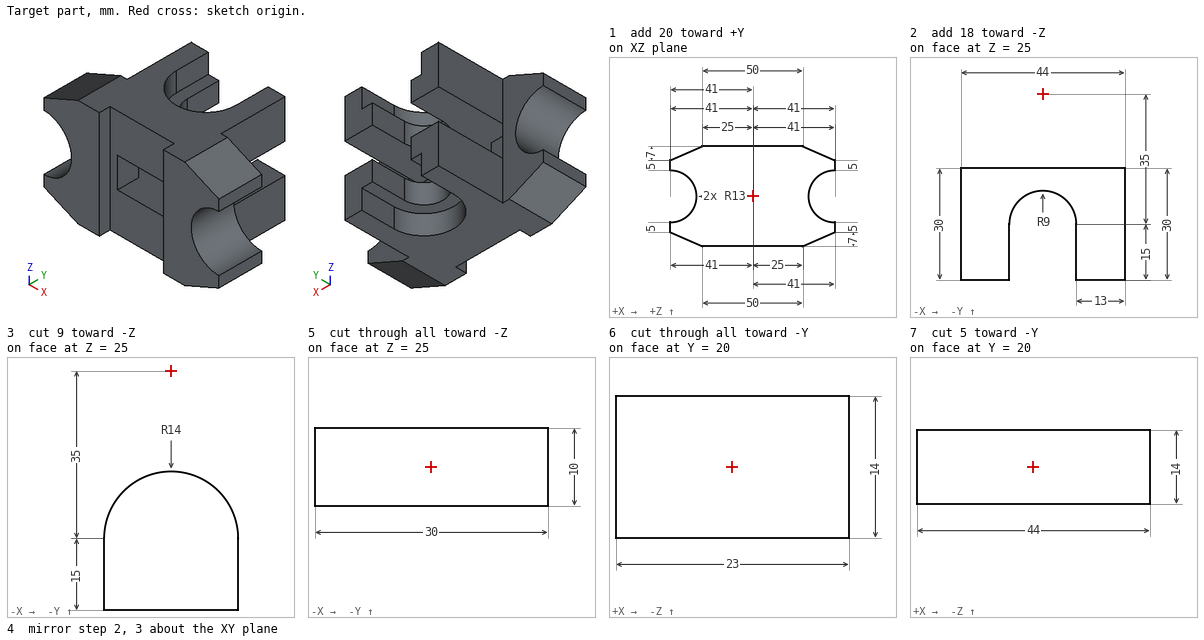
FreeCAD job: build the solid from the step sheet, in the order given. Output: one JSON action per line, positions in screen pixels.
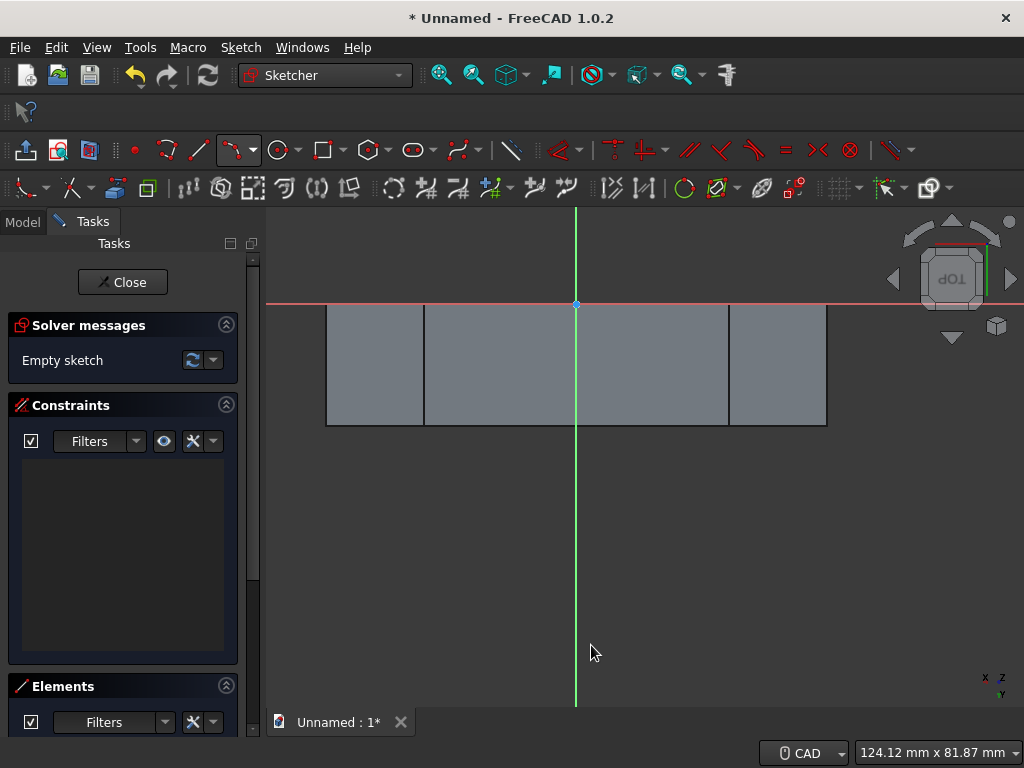
{"action": "left_click", "coordinate": [168, 150]}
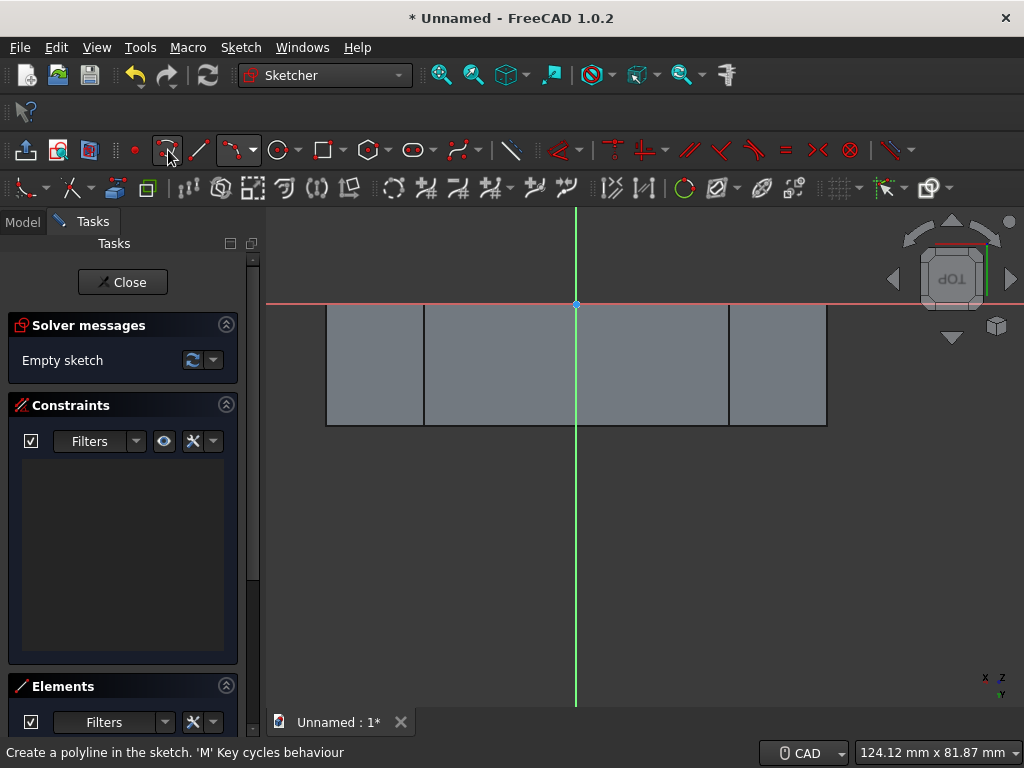
{"action": "left_click", "coordinate": [631, 518]}
{"action": "left_click", "coordinate": [631, 609]}
{"action": "left_click", "coordinate": [711, 609]}
{"action": "left_click", "coordinate": [711, 426]}
{"action": "left_click", "coordinate": [442, 426]}
{"action": "left_click", "coordinate": [442, 609]}
{"action": "left_click", "coordinate": [521, 609]}
{"action": "left_click", "coordinate": [521, 518]}
{"action": "right_click", "coordinate": [521, 518]}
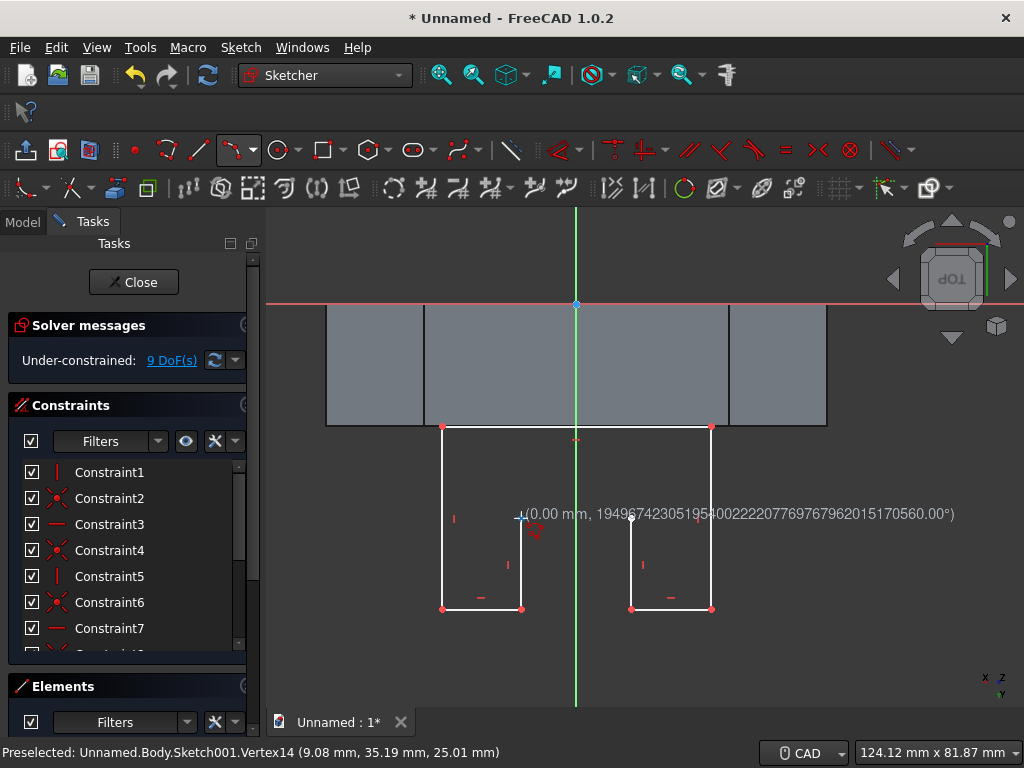
{"action": "left_click", "coordinate": [232, 150]}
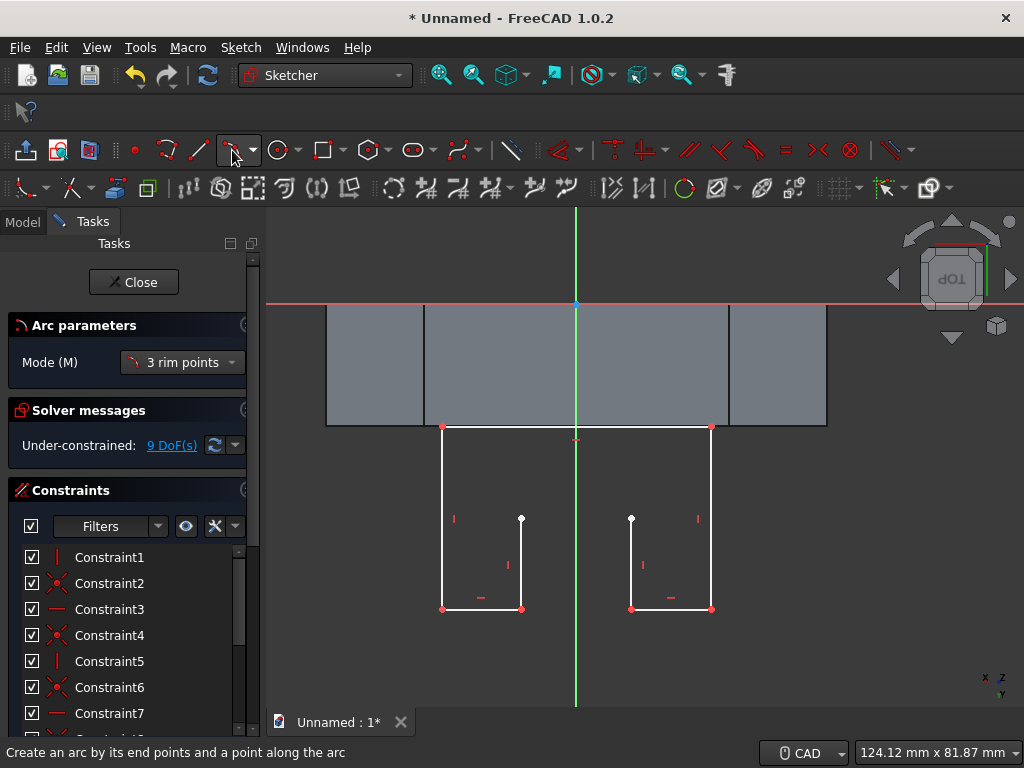
{"action": "left_click", "coordinate": [521, 519]}
{"action": "left_click", "coordinate": [631, 519]}
{"action": "left_click", "coordinate": [593, 466]}
{"action": "key", "text": "Escape"}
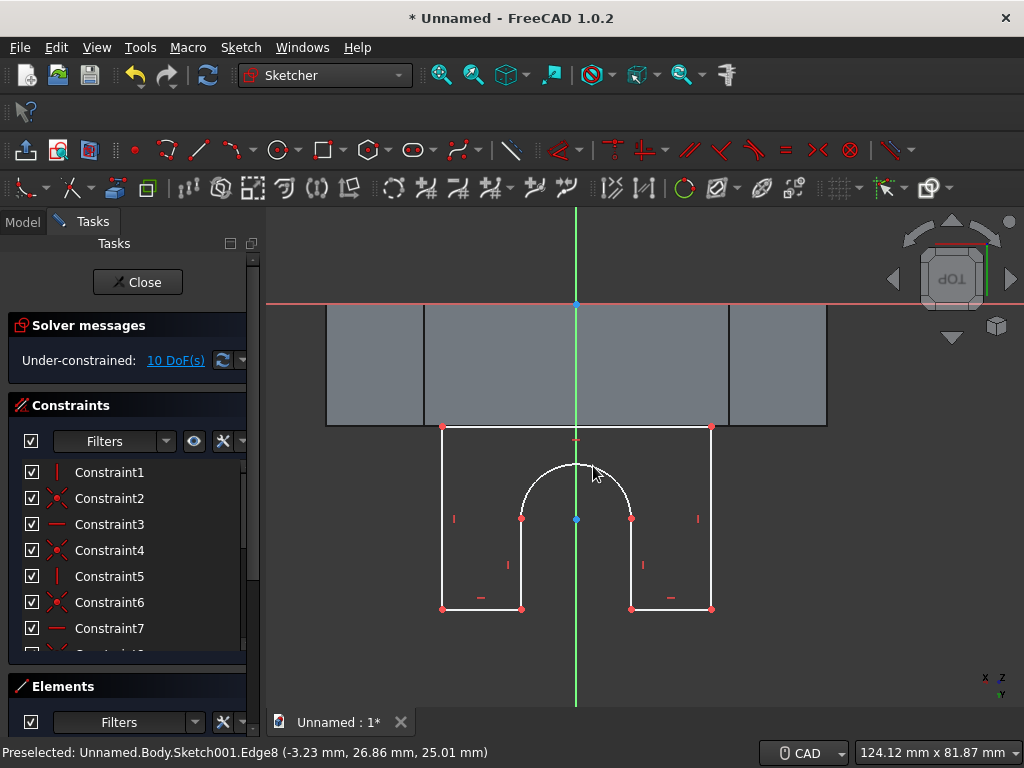
{"action": "left_click", "coordinate": [631, 546]}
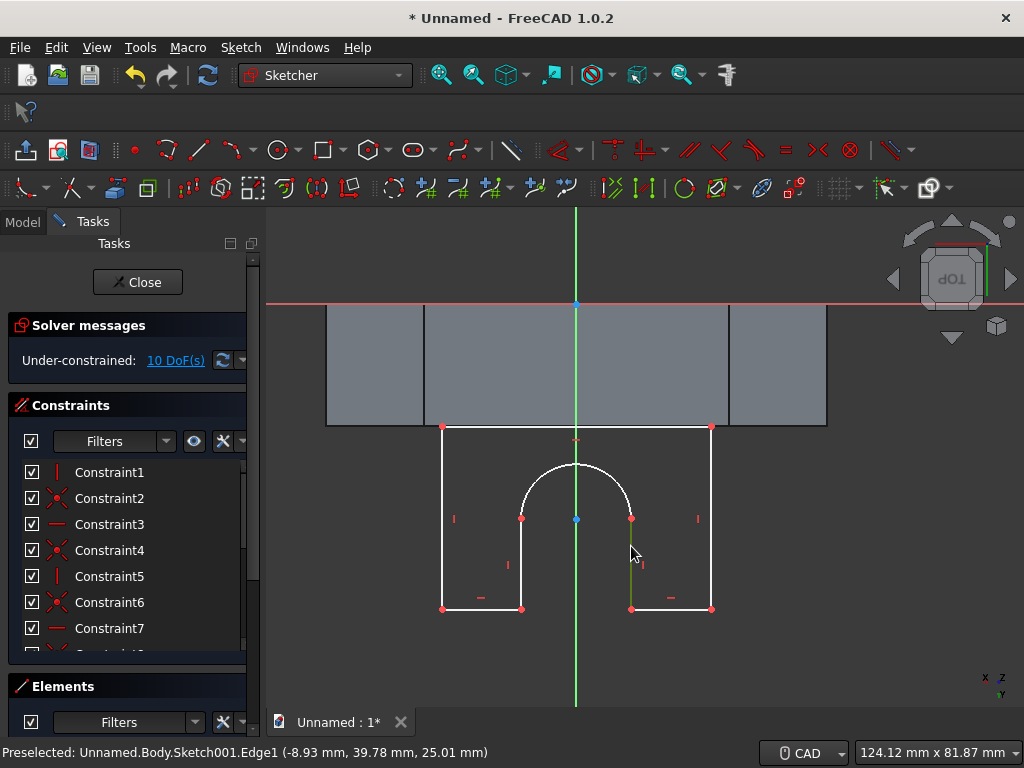
{"action": "left_click", "coordinate": [608, 475]}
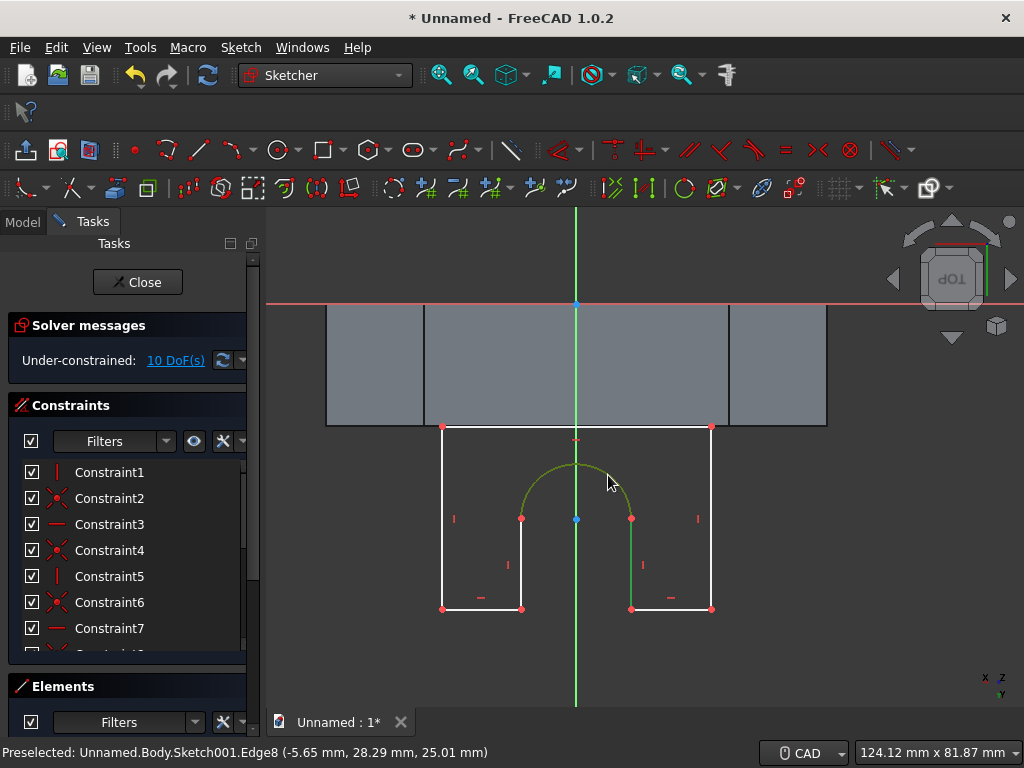
{"action": "left_click", "coordinate": [754, 150]}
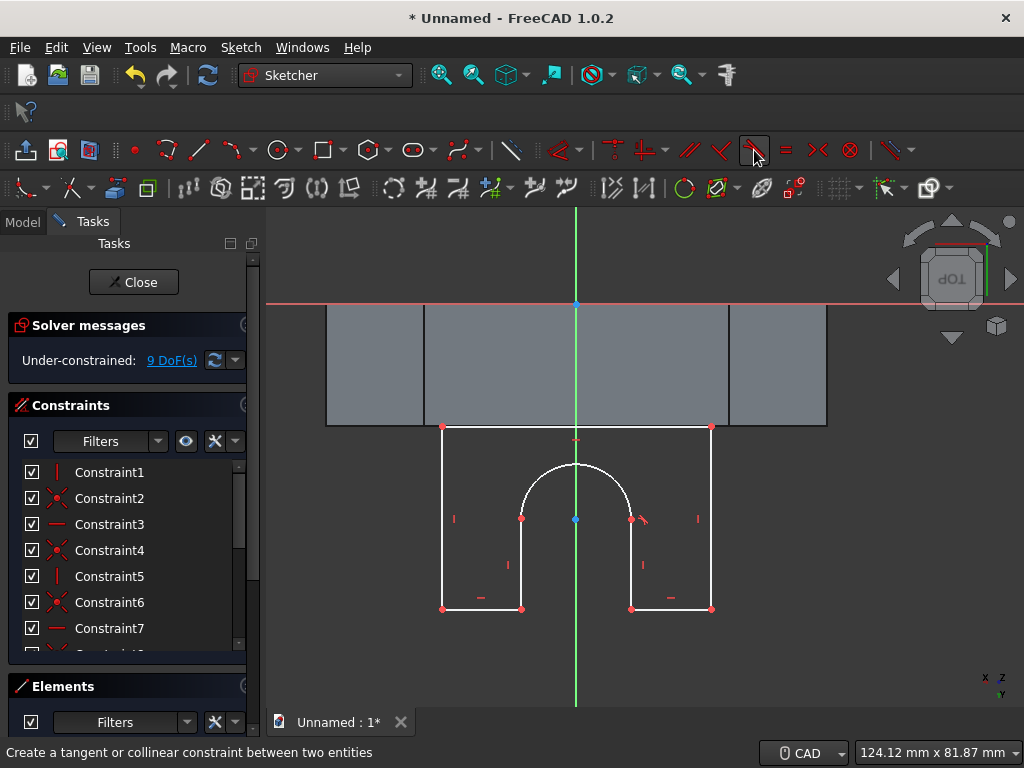
{"action": "left_click", "coordinate": [521, 583]}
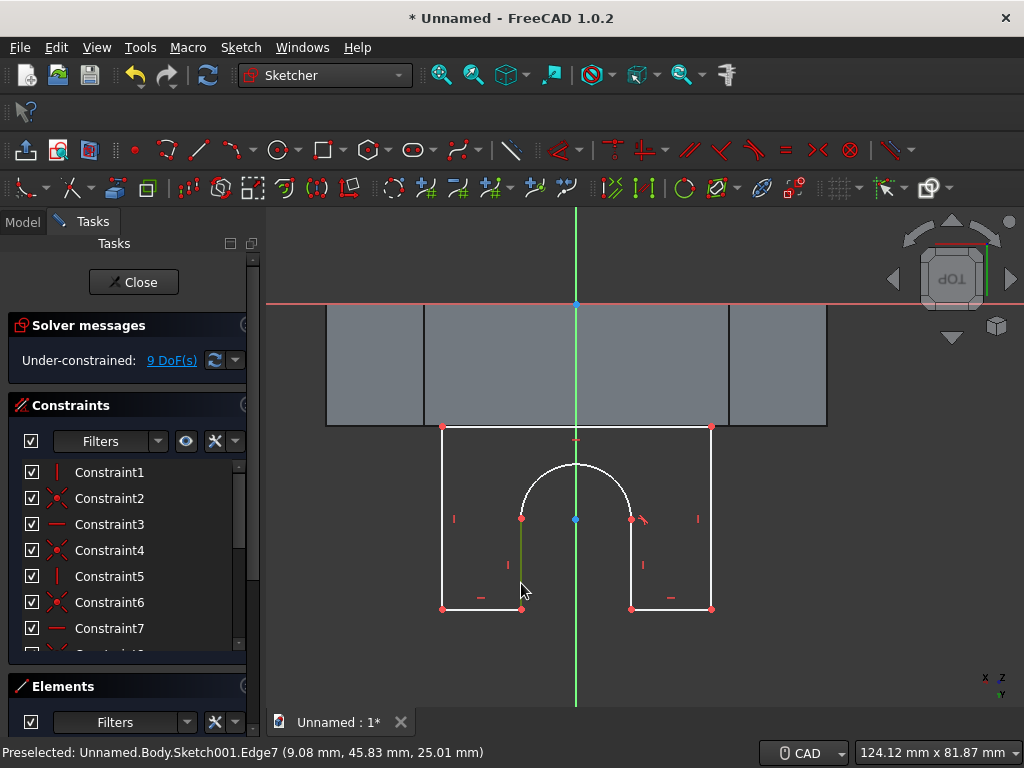
{"action": "left_click", "coordinate": [608, 475]}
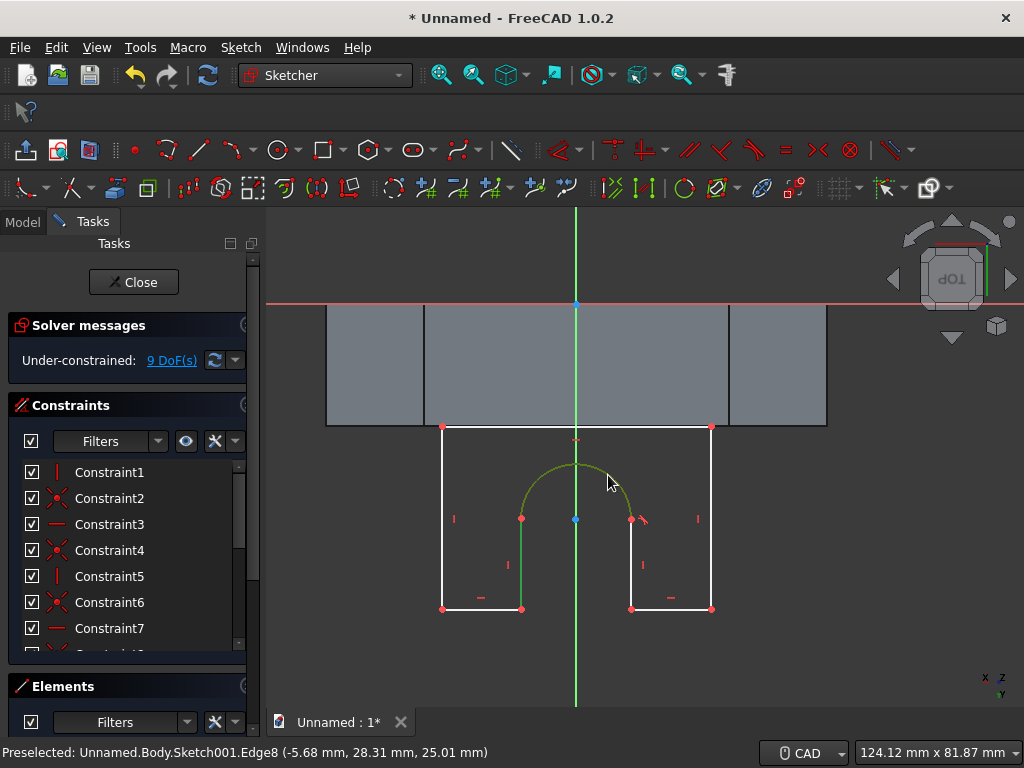
{"action": "left_click", "coordinate": [754, 150]}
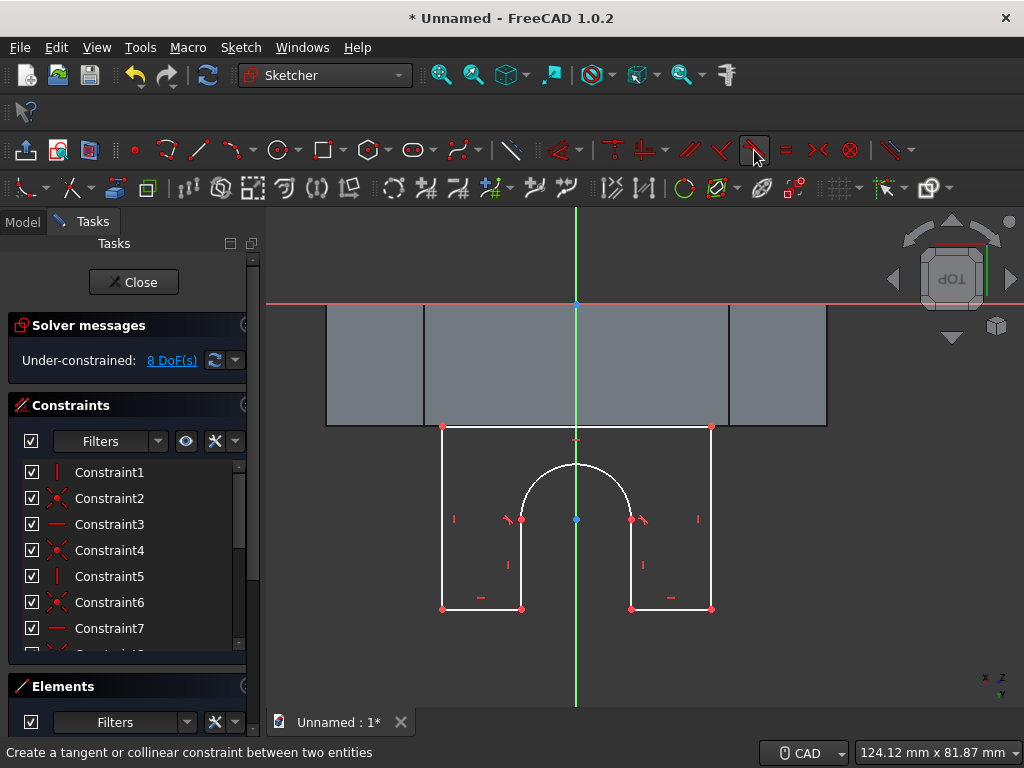
{"action": "left_click", "coordinate": [576, 519]}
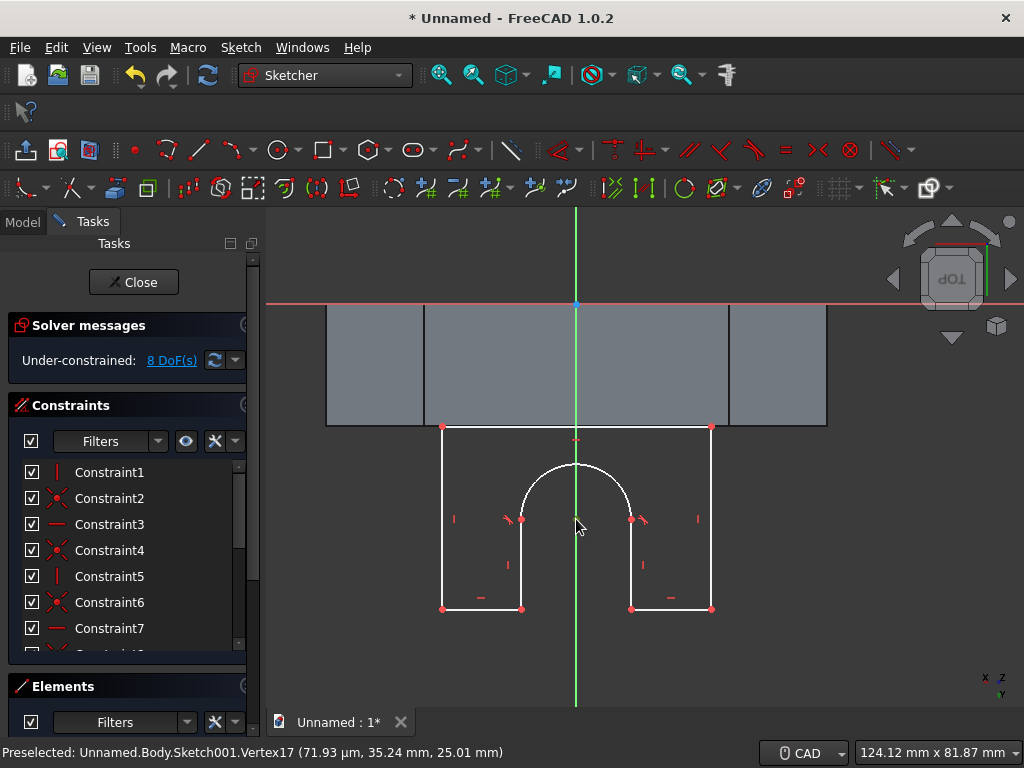
{"action": "left_click", "coordinate": [576, 647]}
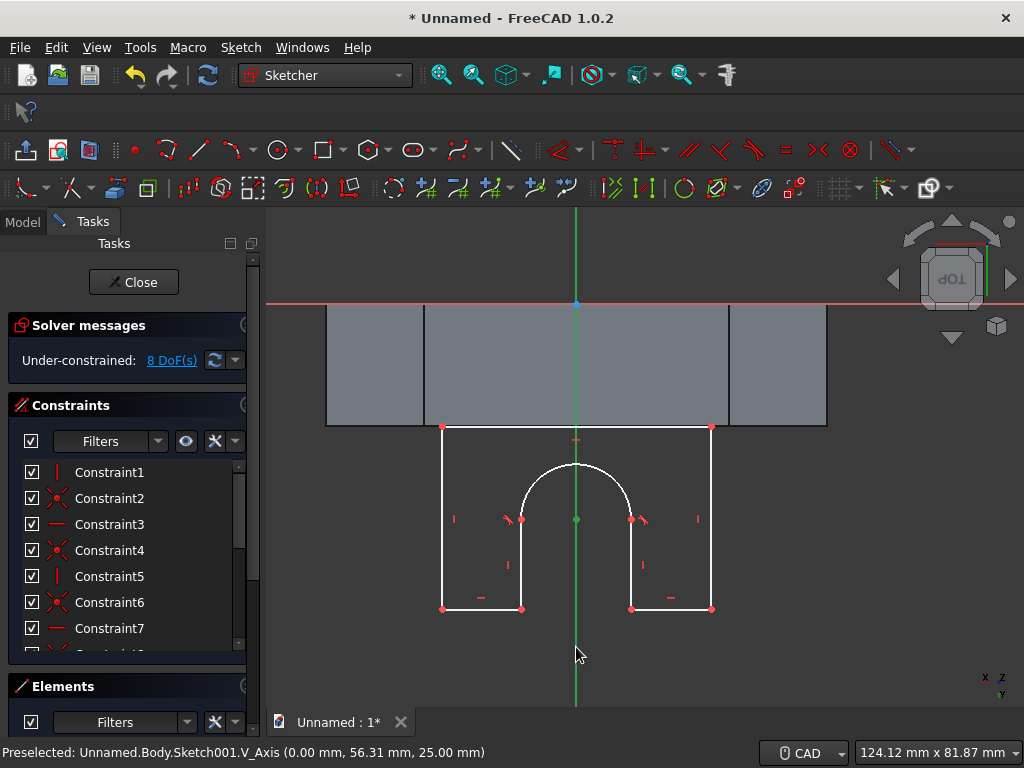
{"action": "left_click", "coordinate": [614, 150]}